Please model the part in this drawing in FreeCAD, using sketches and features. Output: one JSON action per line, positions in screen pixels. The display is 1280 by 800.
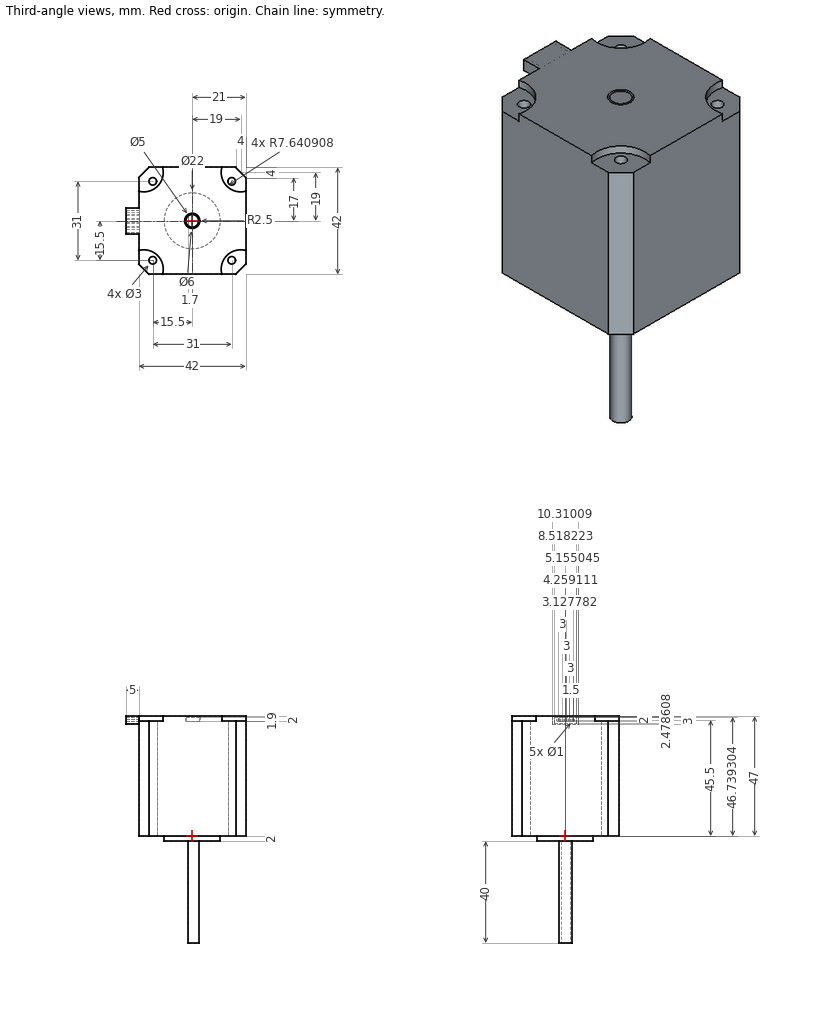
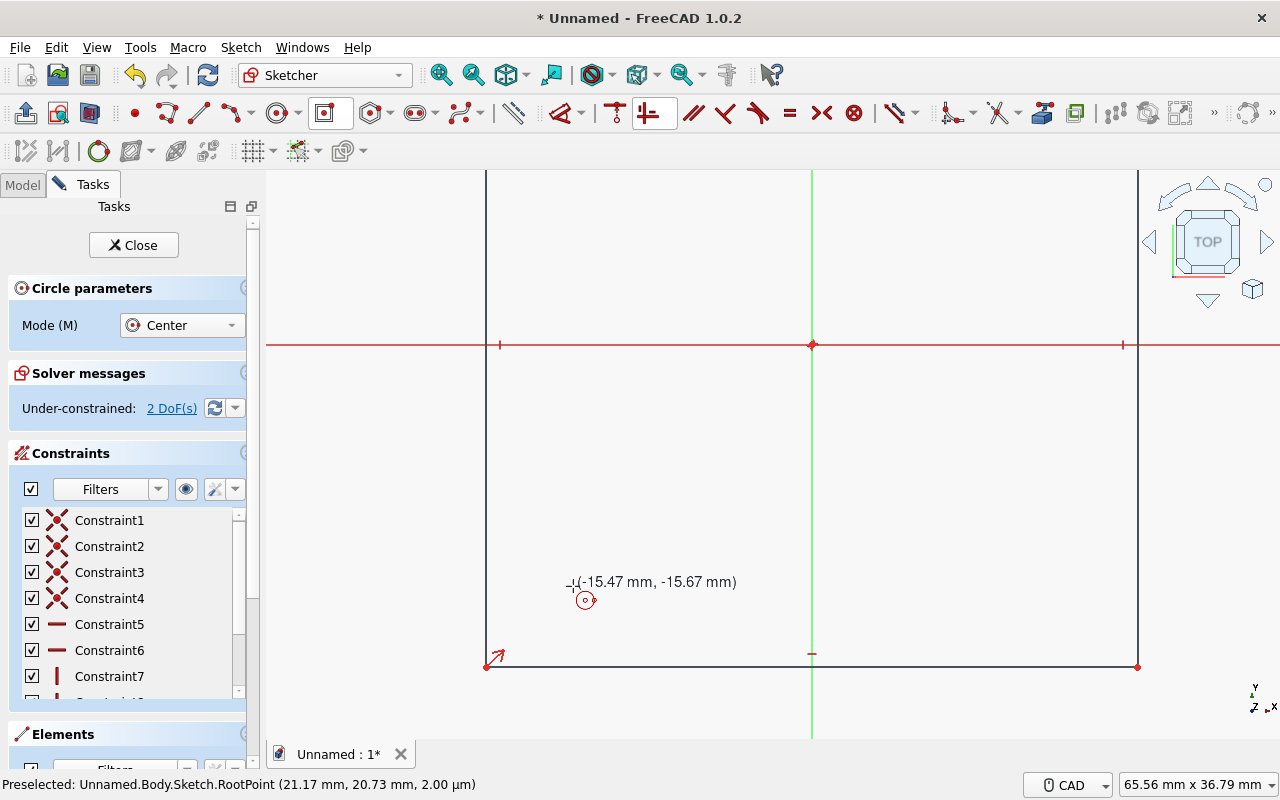
{"action": "left_click", "coordinate": [572, 585]}
{"action": "left_click", "coordinate": [589, 568]}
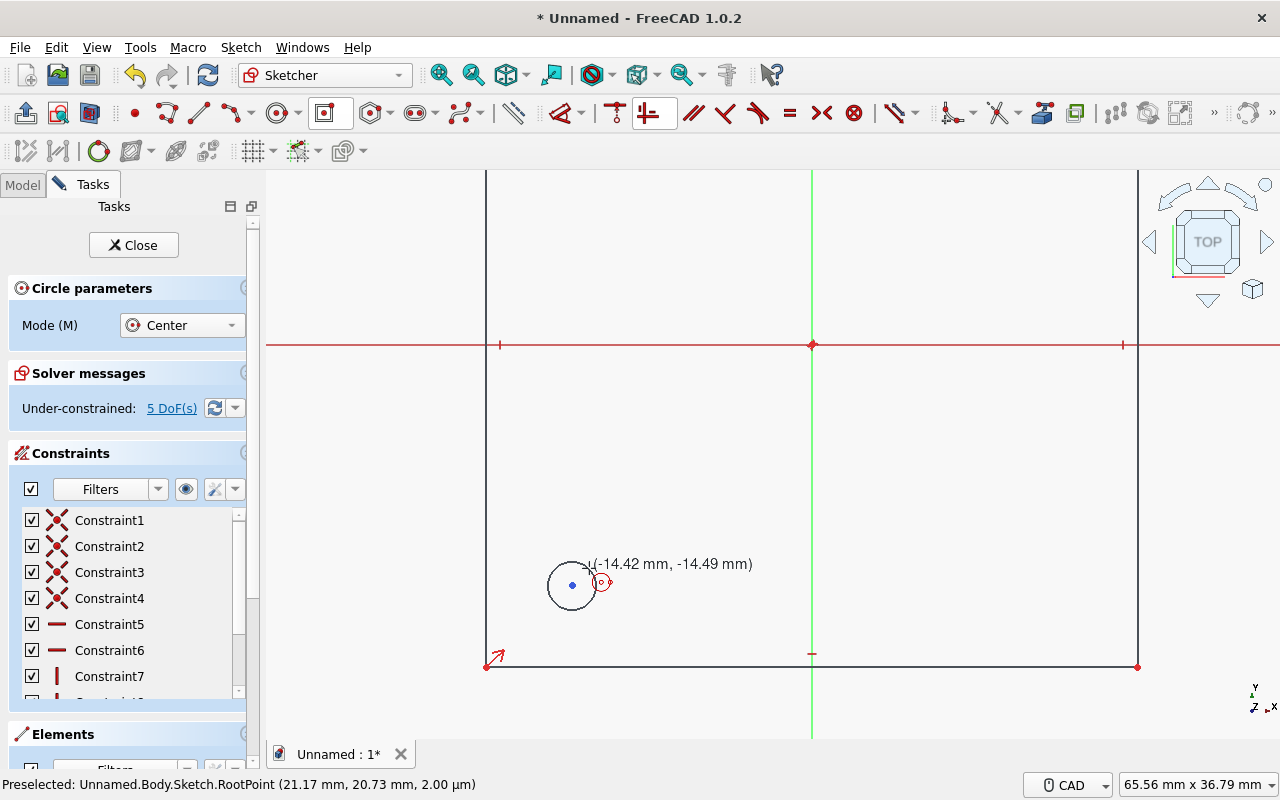
{"action": "left_click", "coordinate": [1052, 585]}
{"action": "left_click", "coordinate": [1068, 568]}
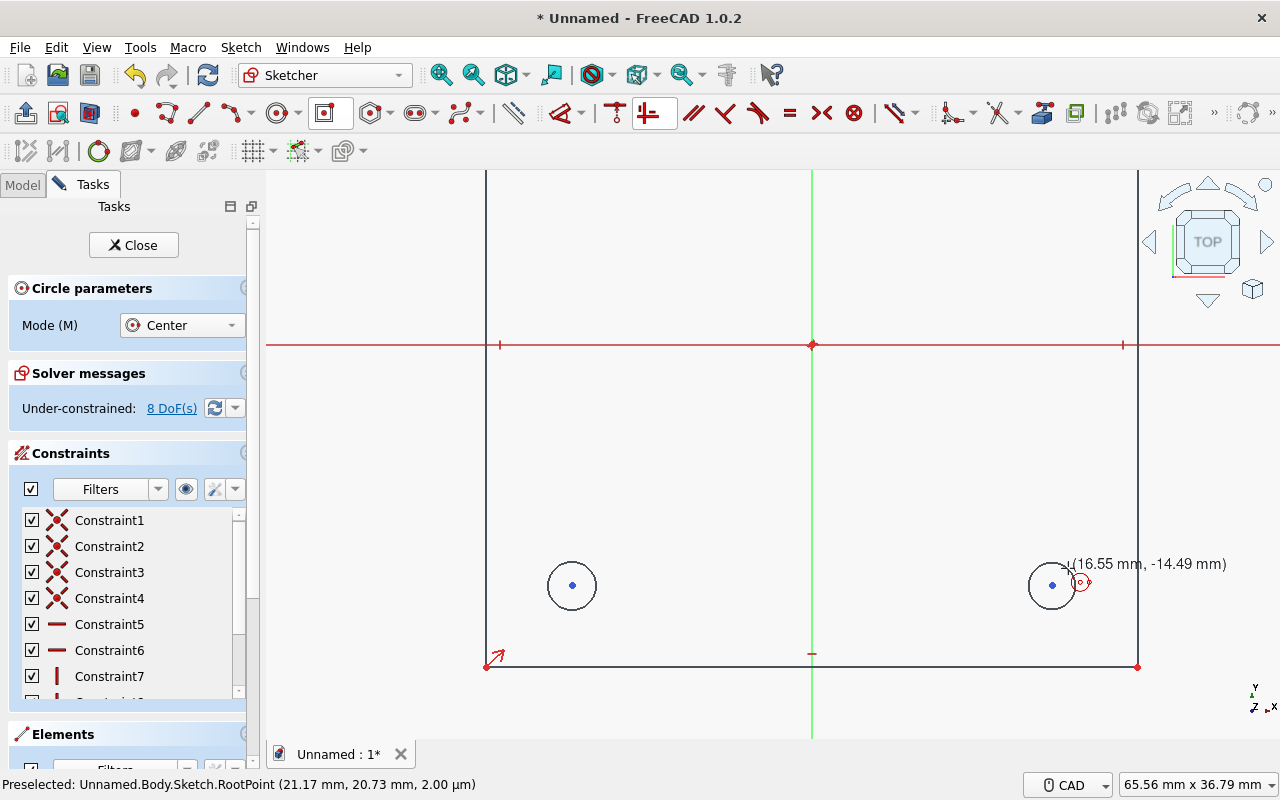
{"action": "scroll", "coordinate": [574, 588], "scroll_direction": "down", "scroll_amount": 3}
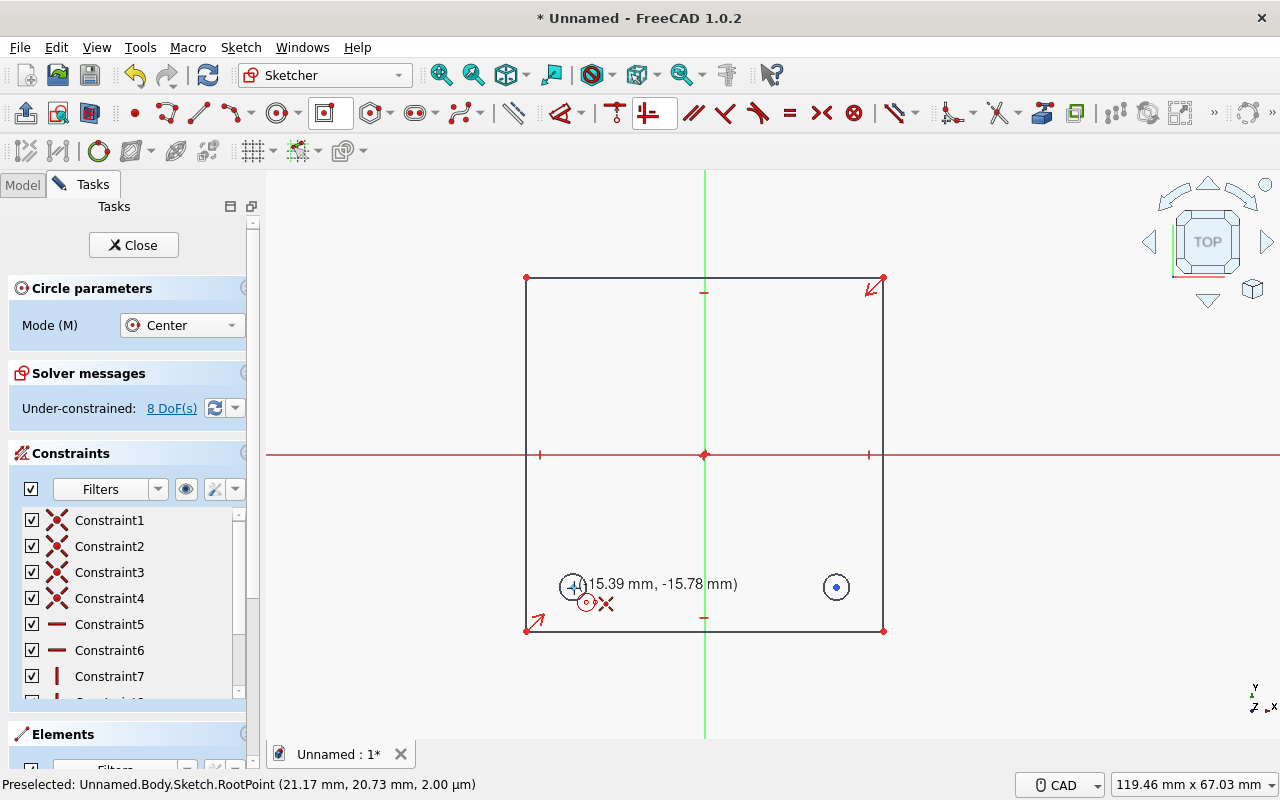
{"action": "scroll", "coordinate": [573, 323], "scroll_direction": "up", "scroll_amount": 3}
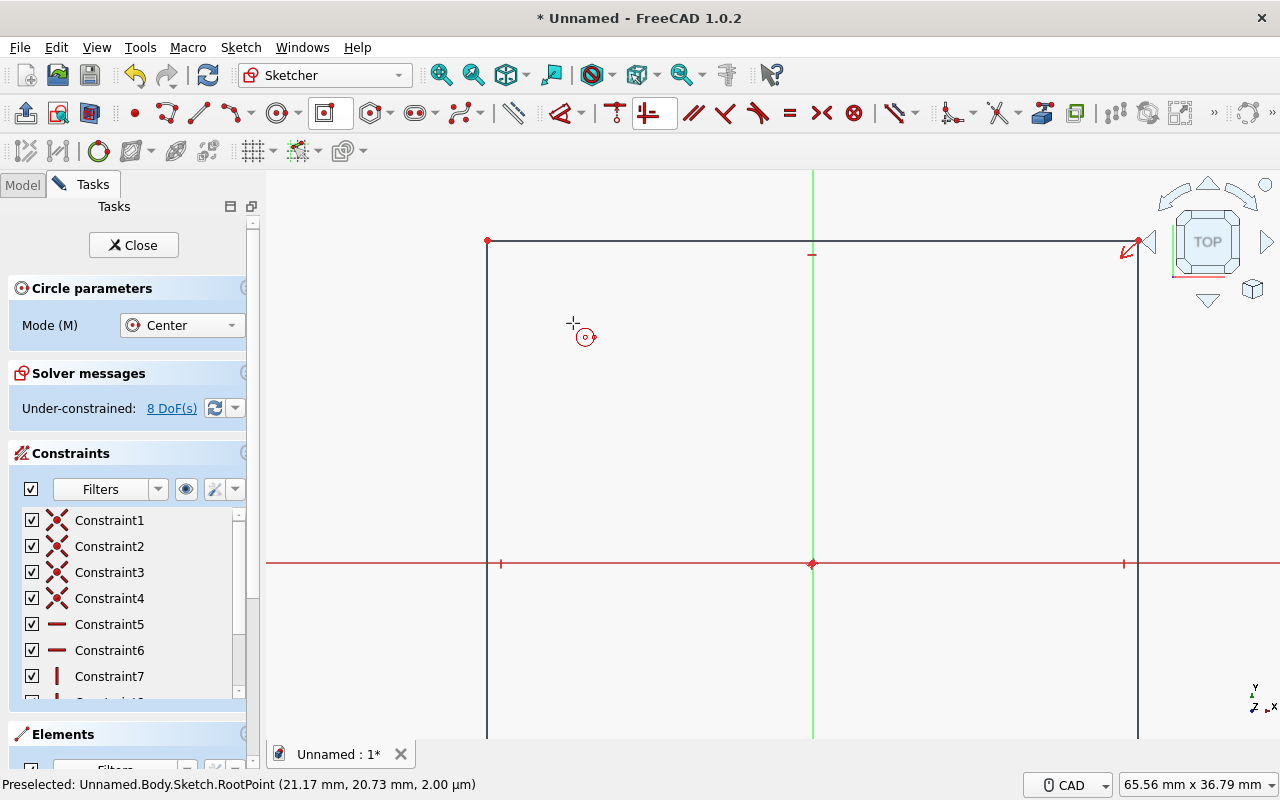
{"action": "left_click", "coordinate": [573, 323]}
{"action": "left_click", "coordinate": [590, 307]}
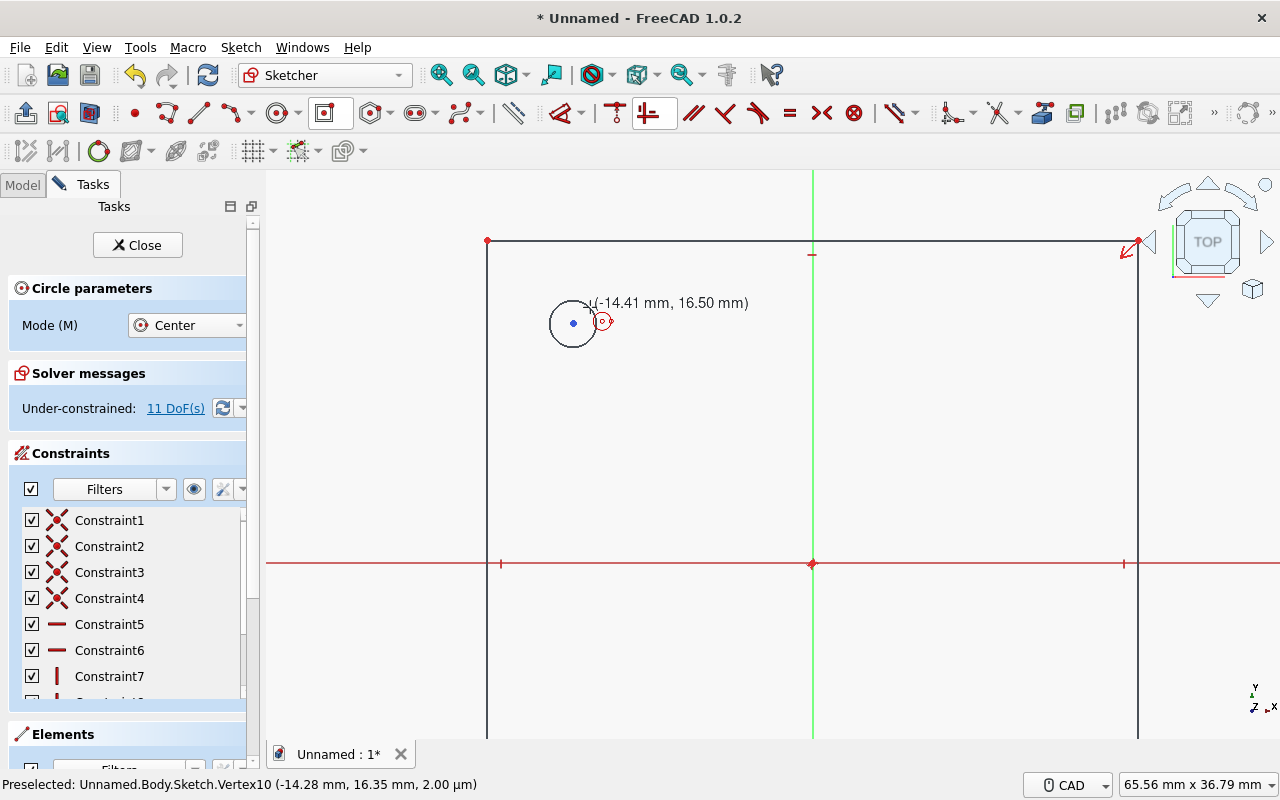
{"action": "left_click", "coordinate": [1053, 323]}
{"action": "left_click", "coordinate": [1069, 307]}
{"action": "key", "text": "Escape"}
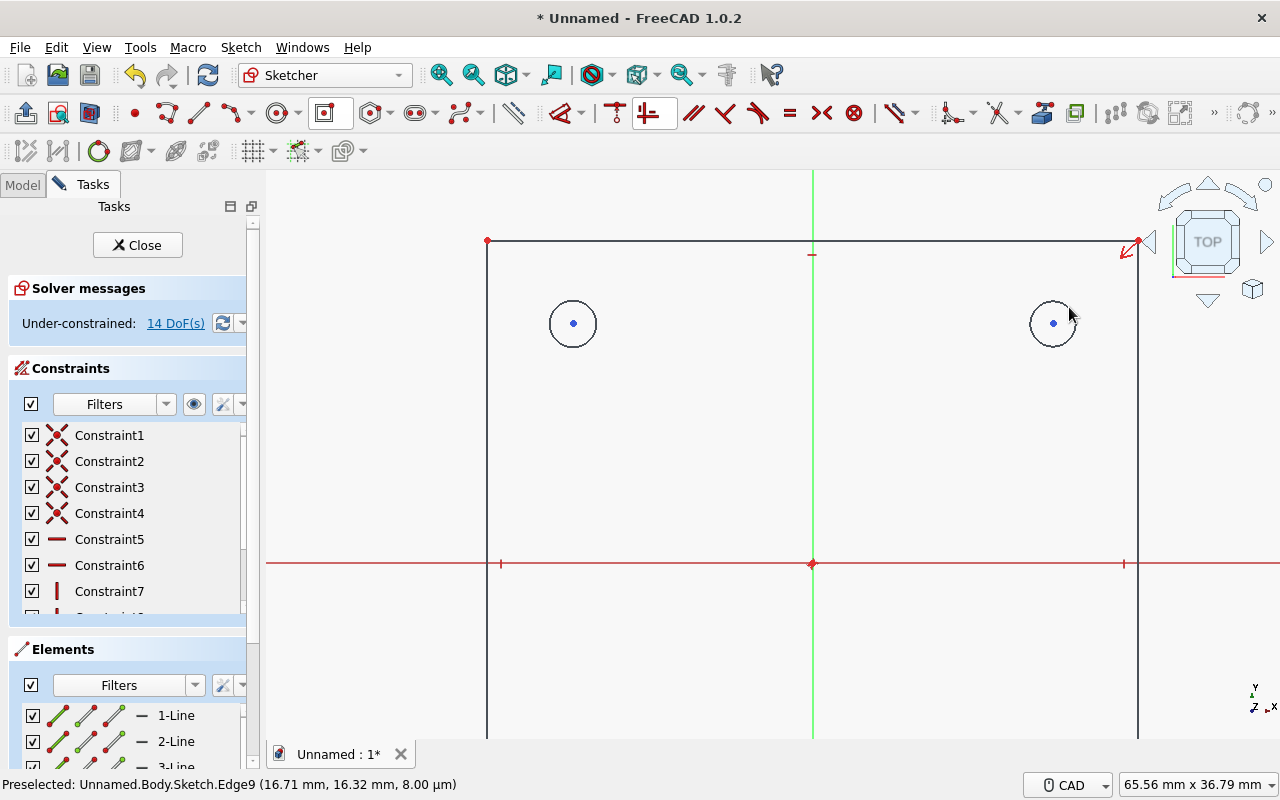
{"action": "scroll", "coordinate": [573, 322], "scroll_direction": "down", "scroll_amount": 3}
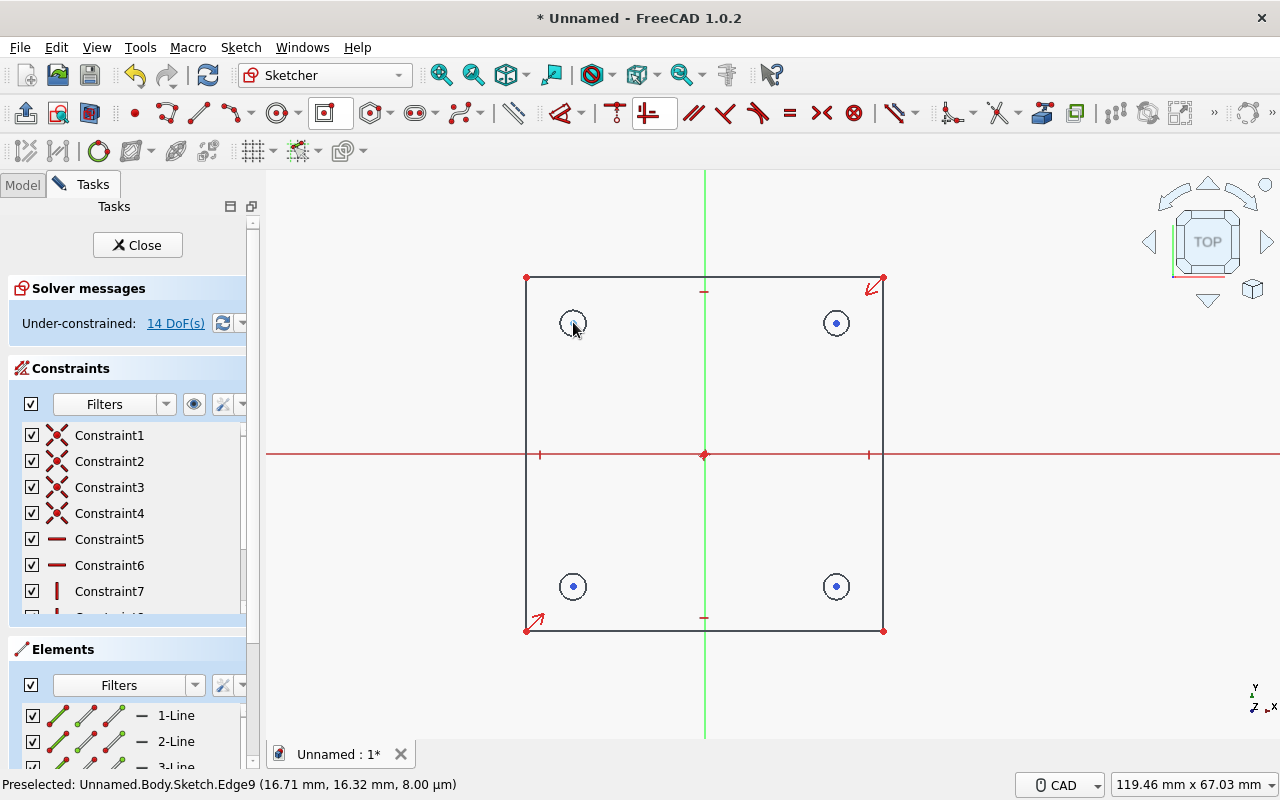
{"action": "left_click", "coordinate": [582, 577]}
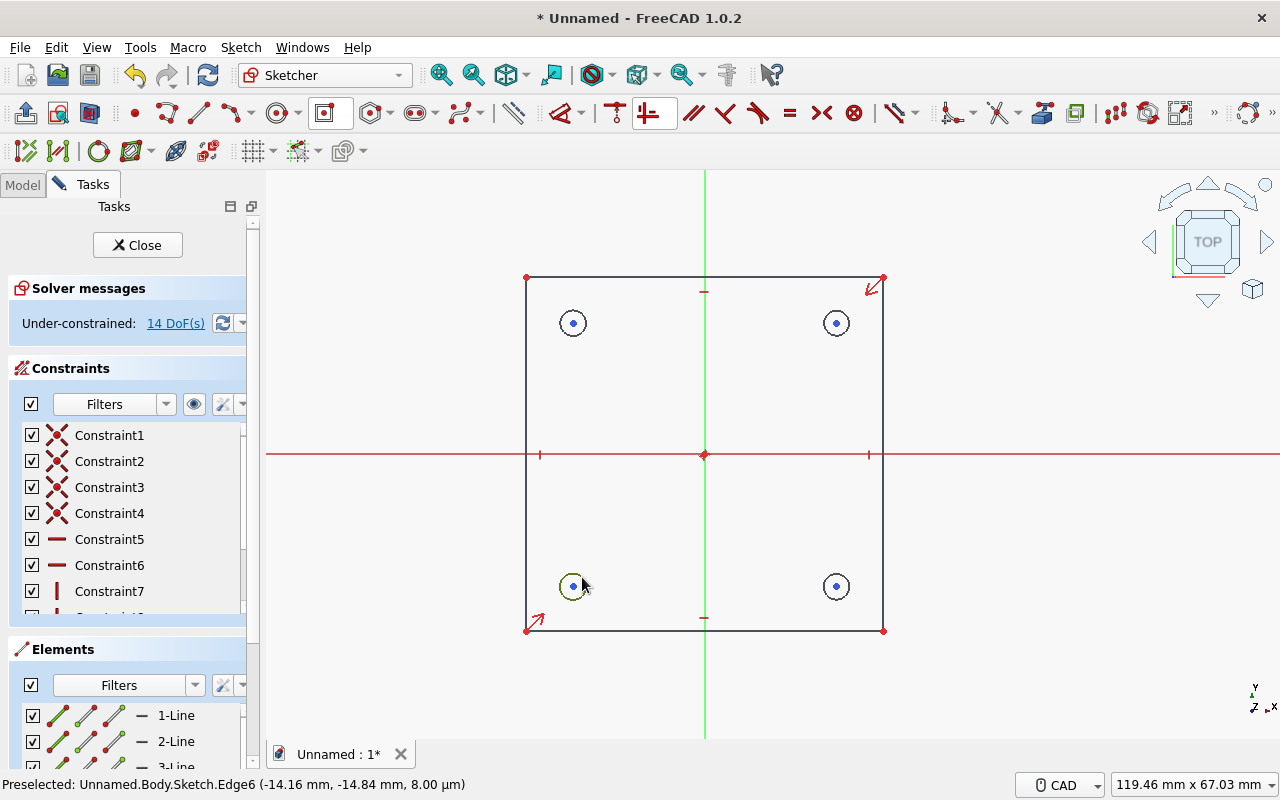
{"action": "left_click", "coordinate": [846, 578]}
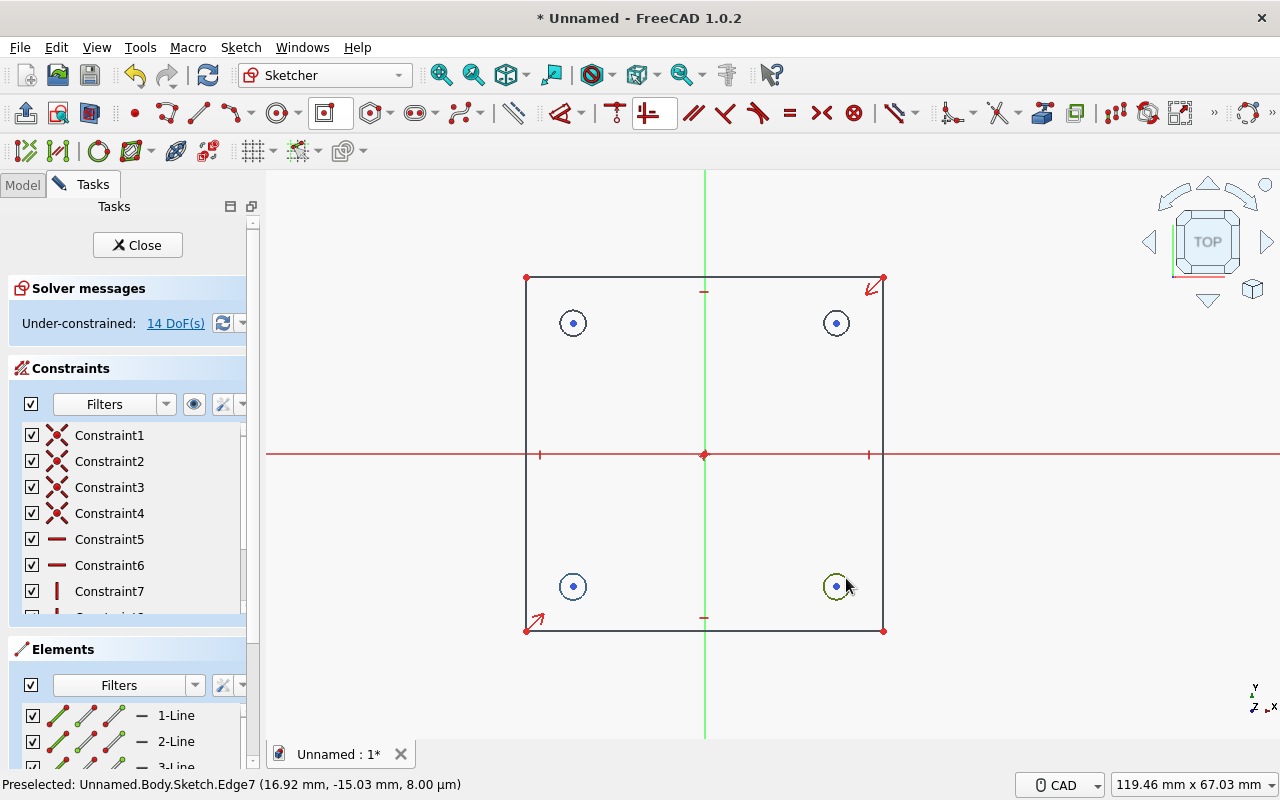
{"action": "left_click", "coordinate": [582, 314]}